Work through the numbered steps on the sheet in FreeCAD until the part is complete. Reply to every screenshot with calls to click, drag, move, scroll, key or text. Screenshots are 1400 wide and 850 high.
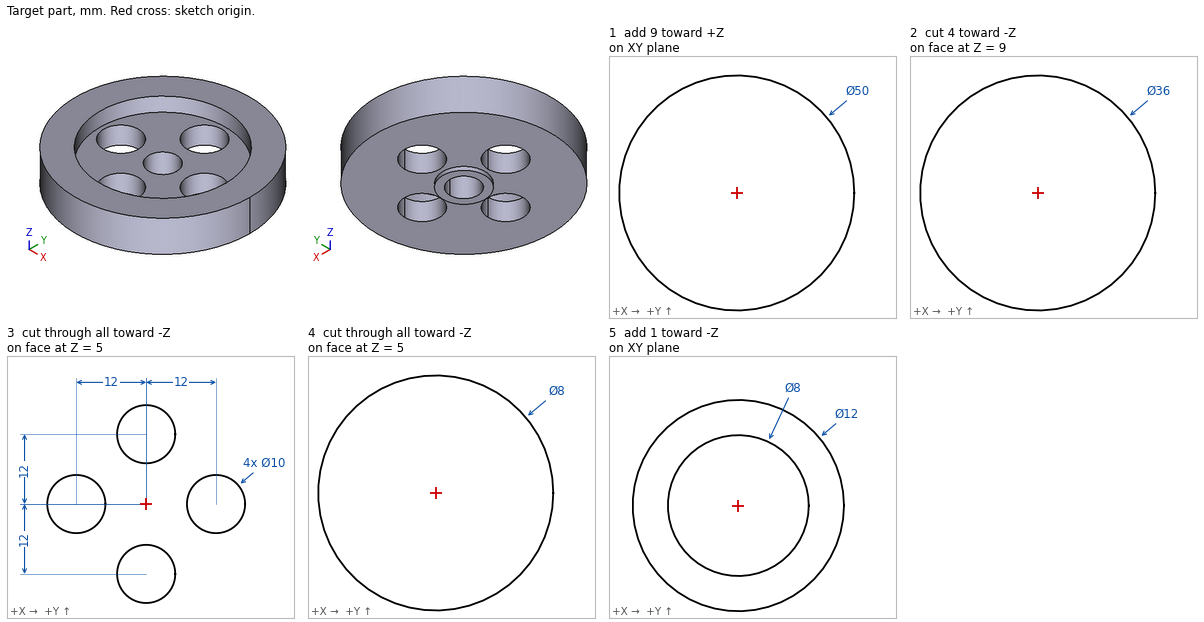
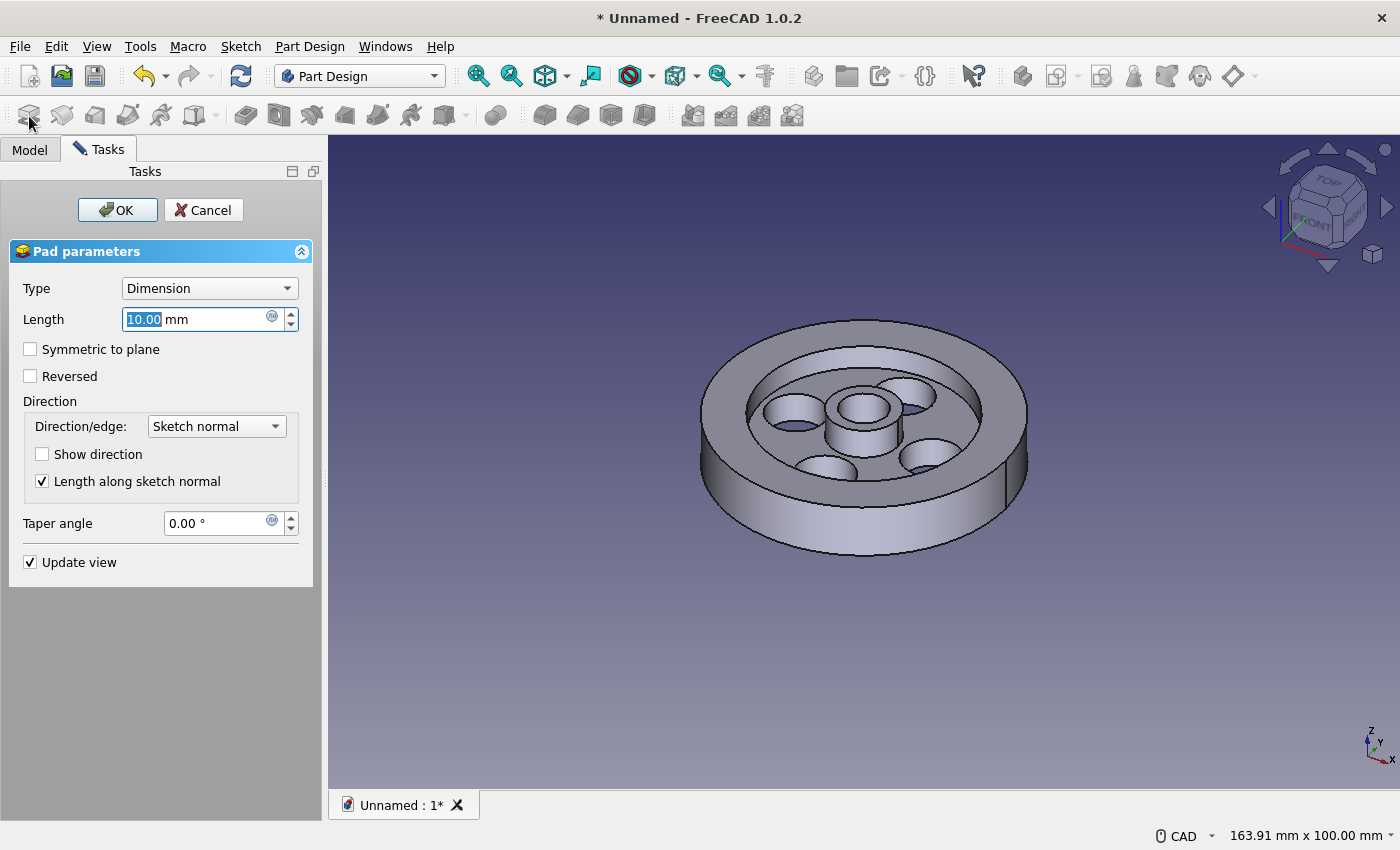
text(1)
key(Tab)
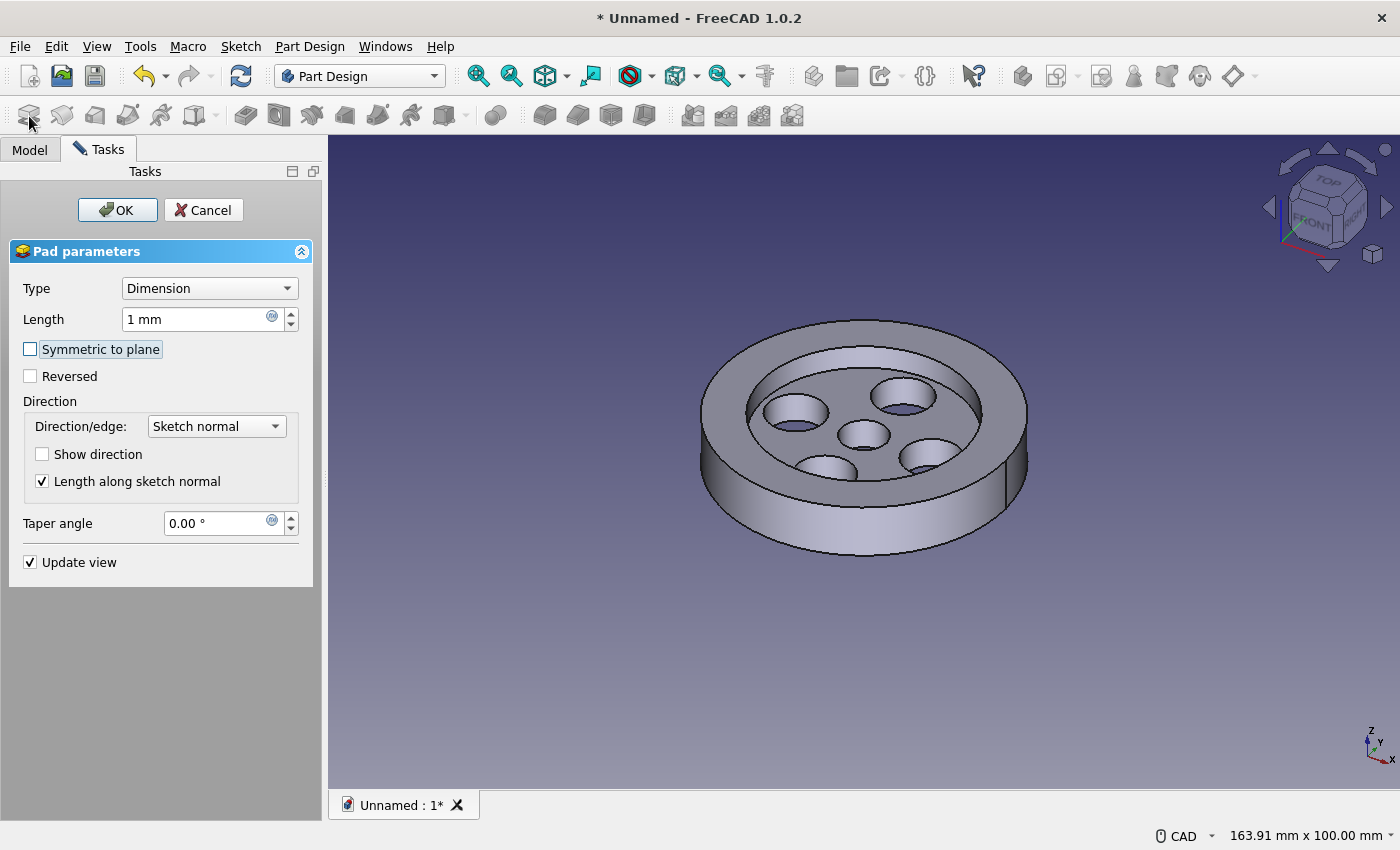
click(31, 376)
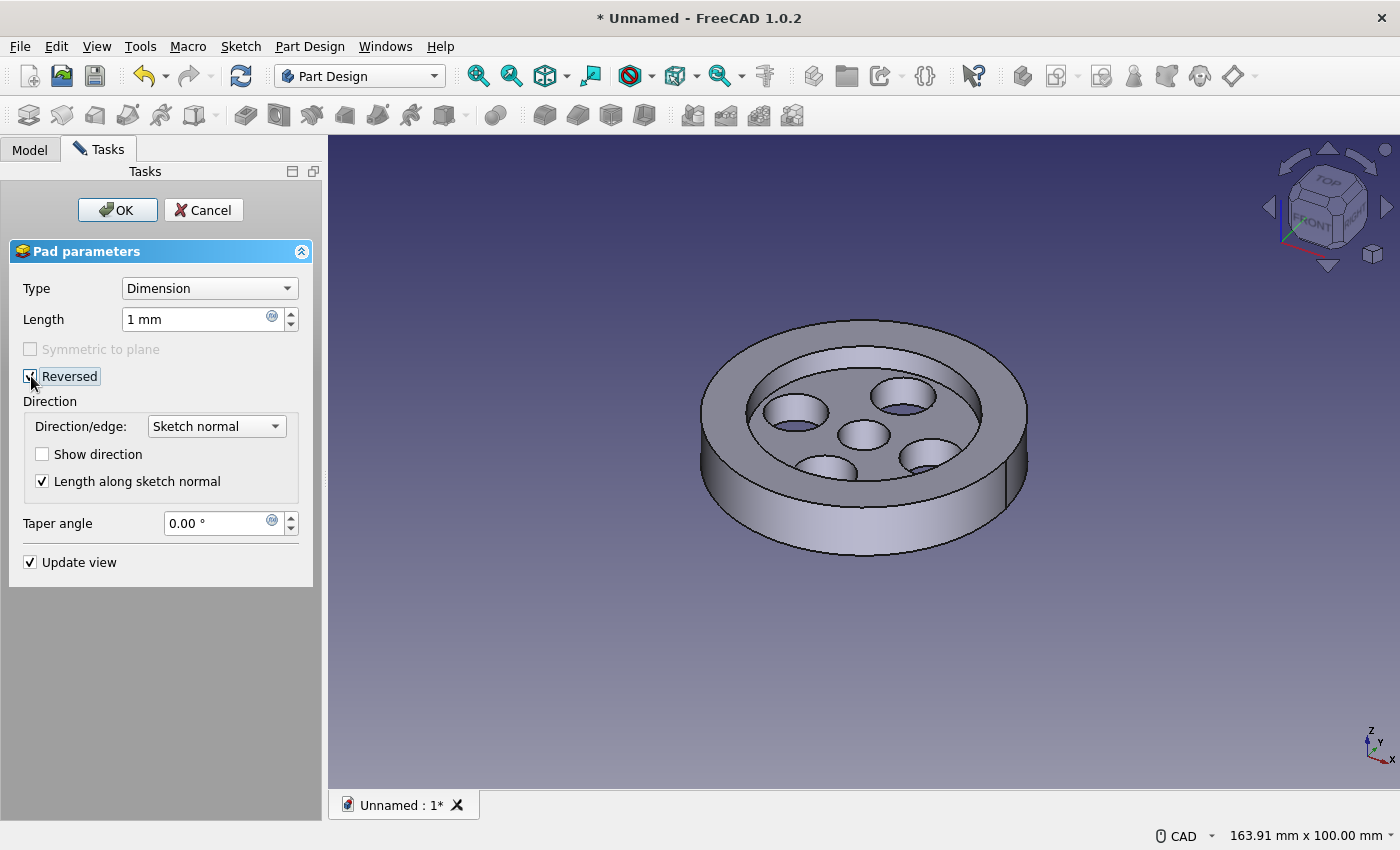
click(118, 210)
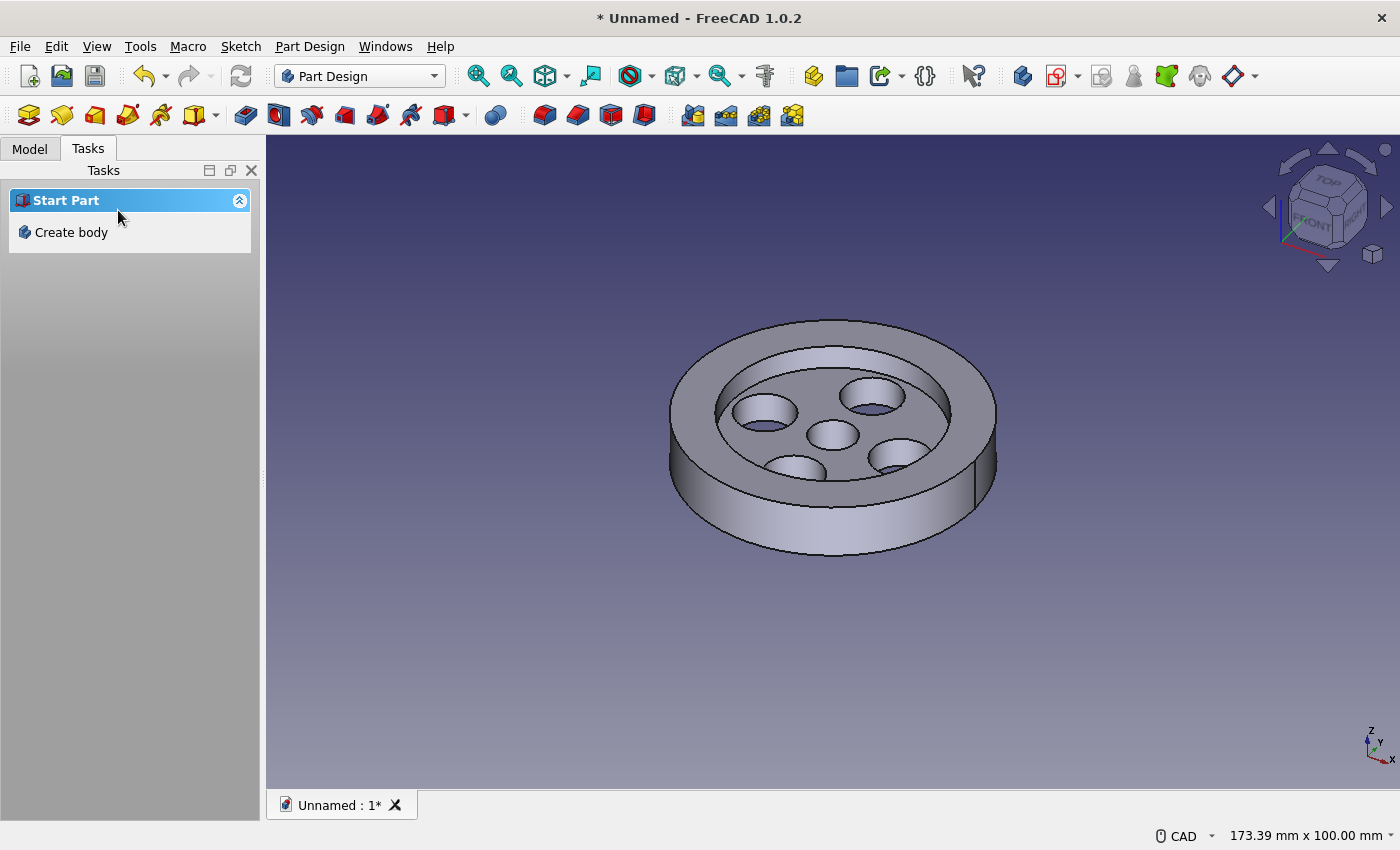
key(0)